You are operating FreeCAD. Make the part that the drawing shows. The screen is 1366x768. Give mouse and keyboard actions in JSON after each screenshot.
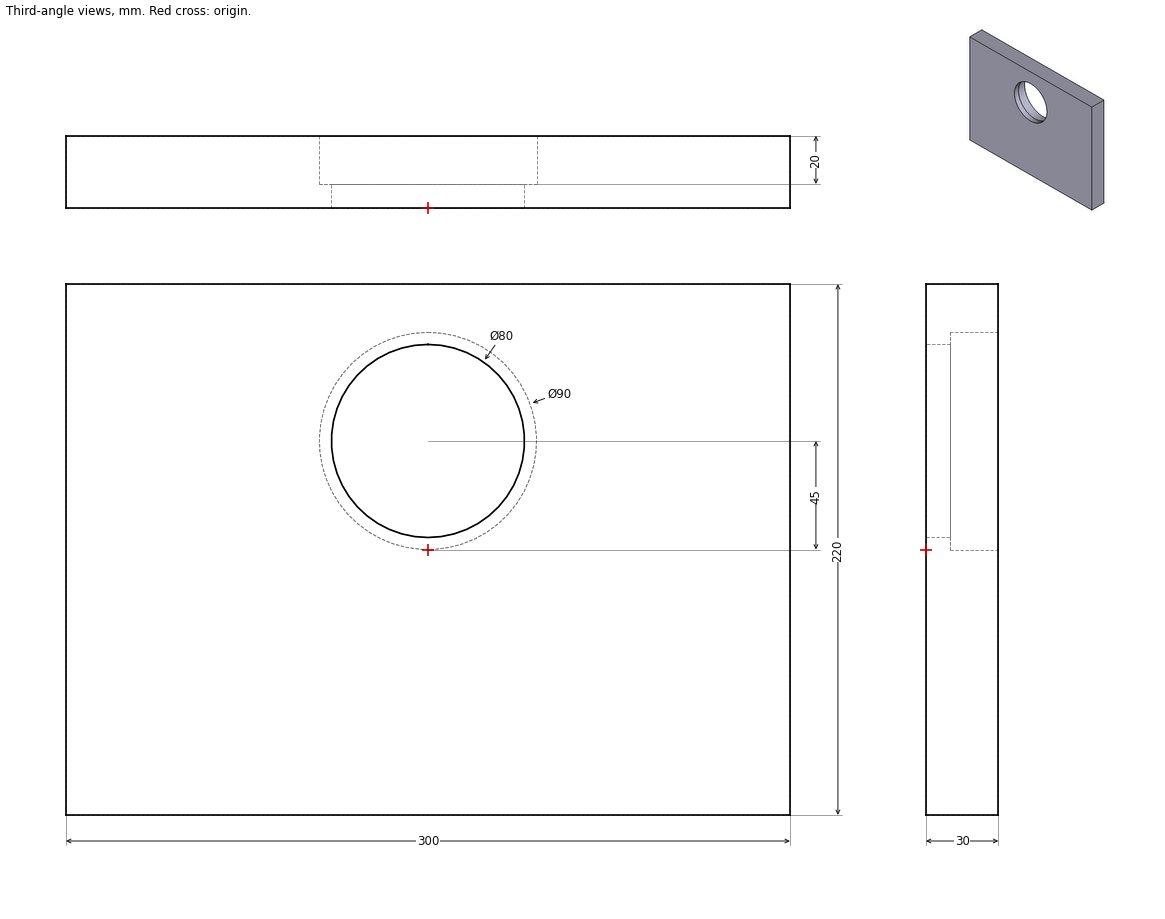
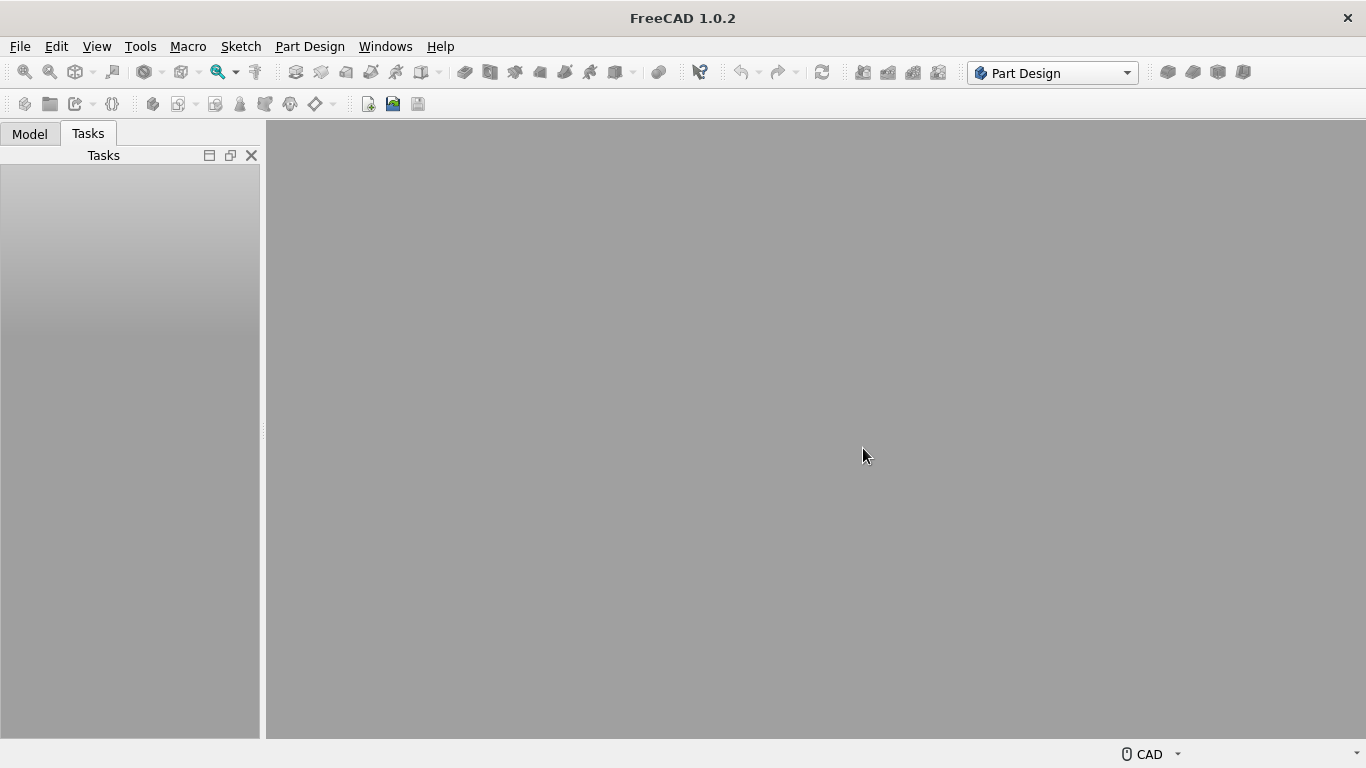
{"action": "left_click", "coordinate": [368, 104]}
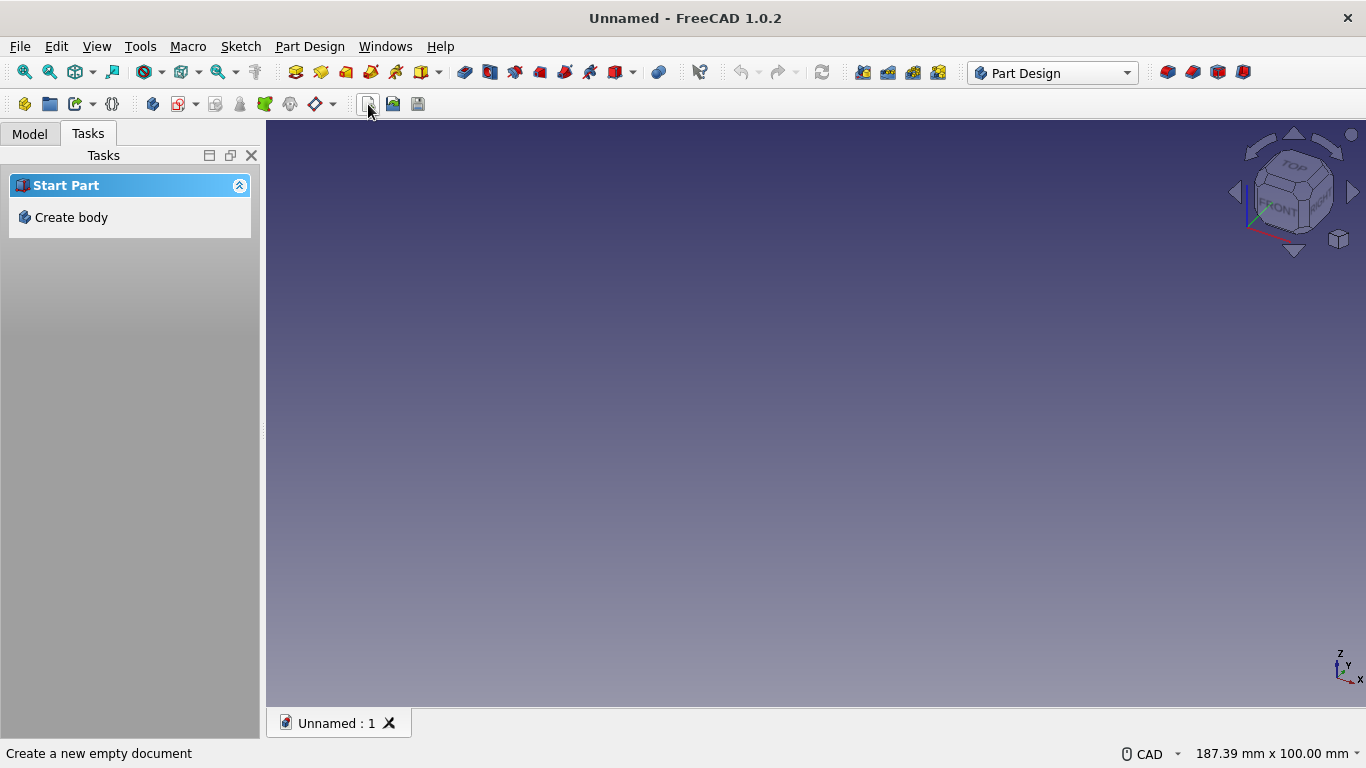
{"action": "left_click", "coordinate": [178, 104]}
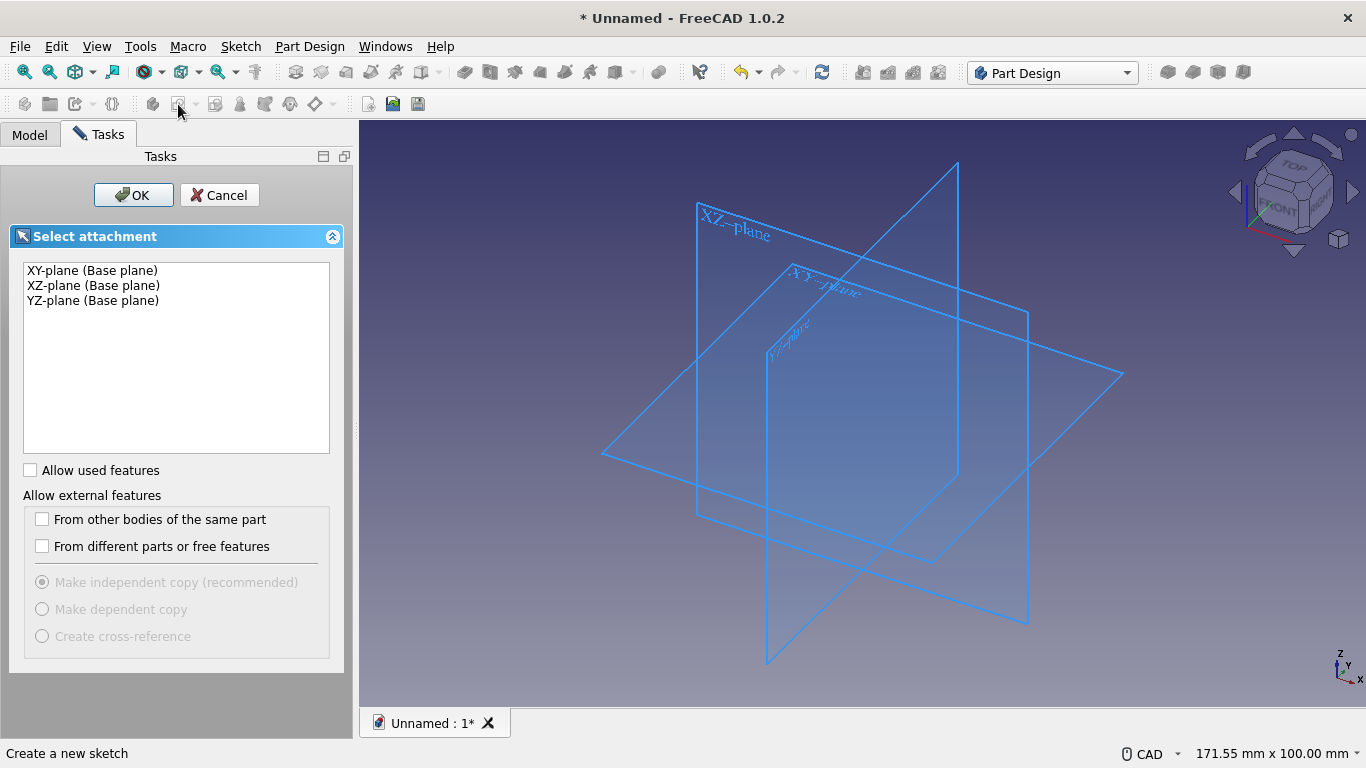
{"action": "left_click", "coordinate": [84, 286]}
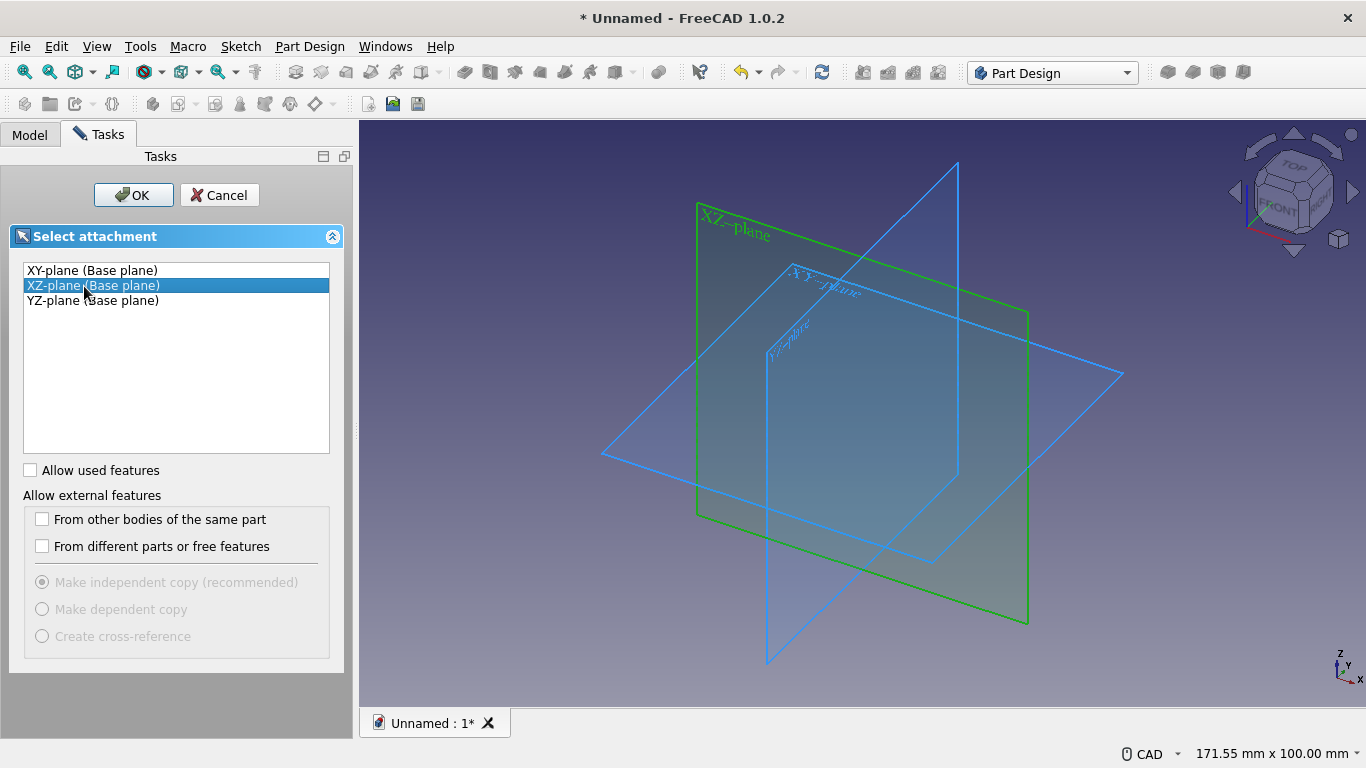
{"action": "left_click", "coordinate": [134, 195]}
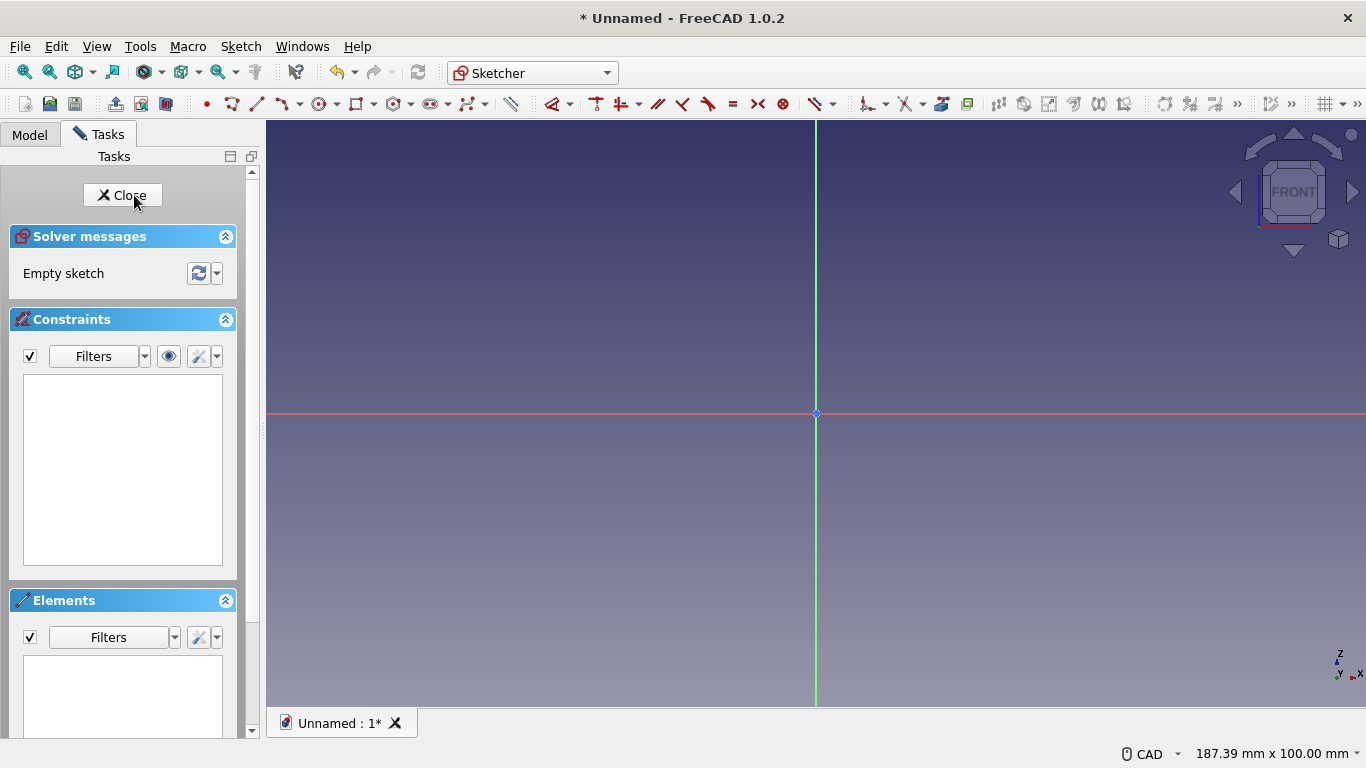
{"action": "scroll", "coordinate": [718, 413], "scroll_direction": "down", "scroll_amount": 6}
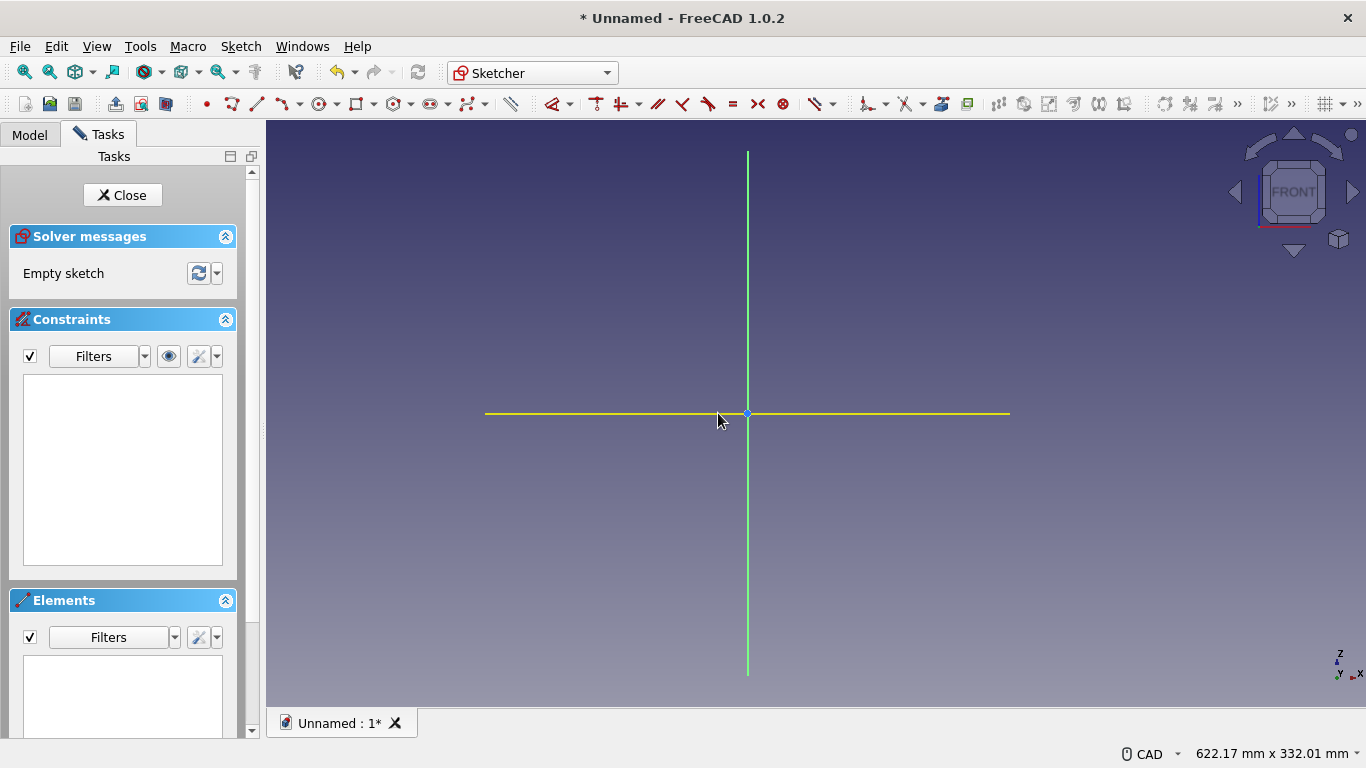
{"action": "key", "text": "g v"}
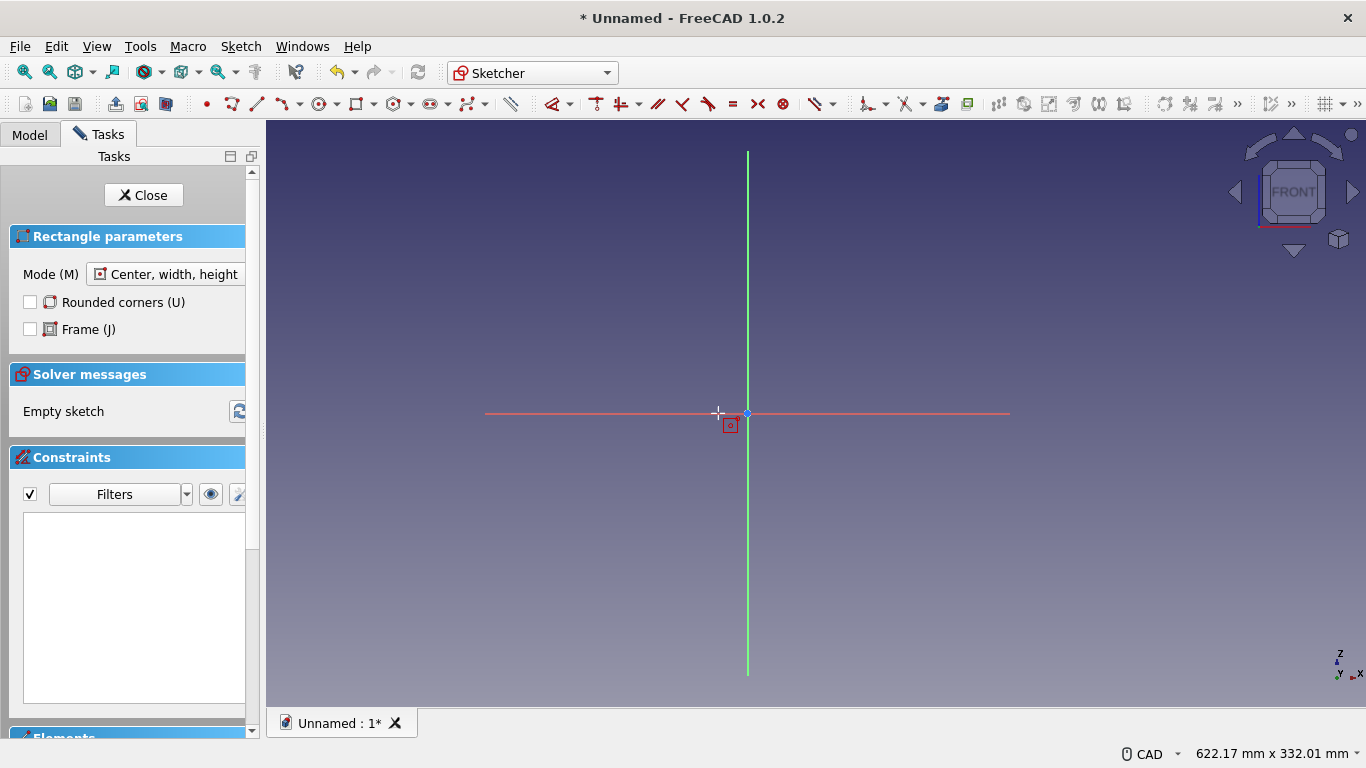
{"action": "left_click", "coordinate": [748, 414]}
{"action": "left_click", "coordinate": [1013, 219]}
{"action": "key", "text": "Escape"}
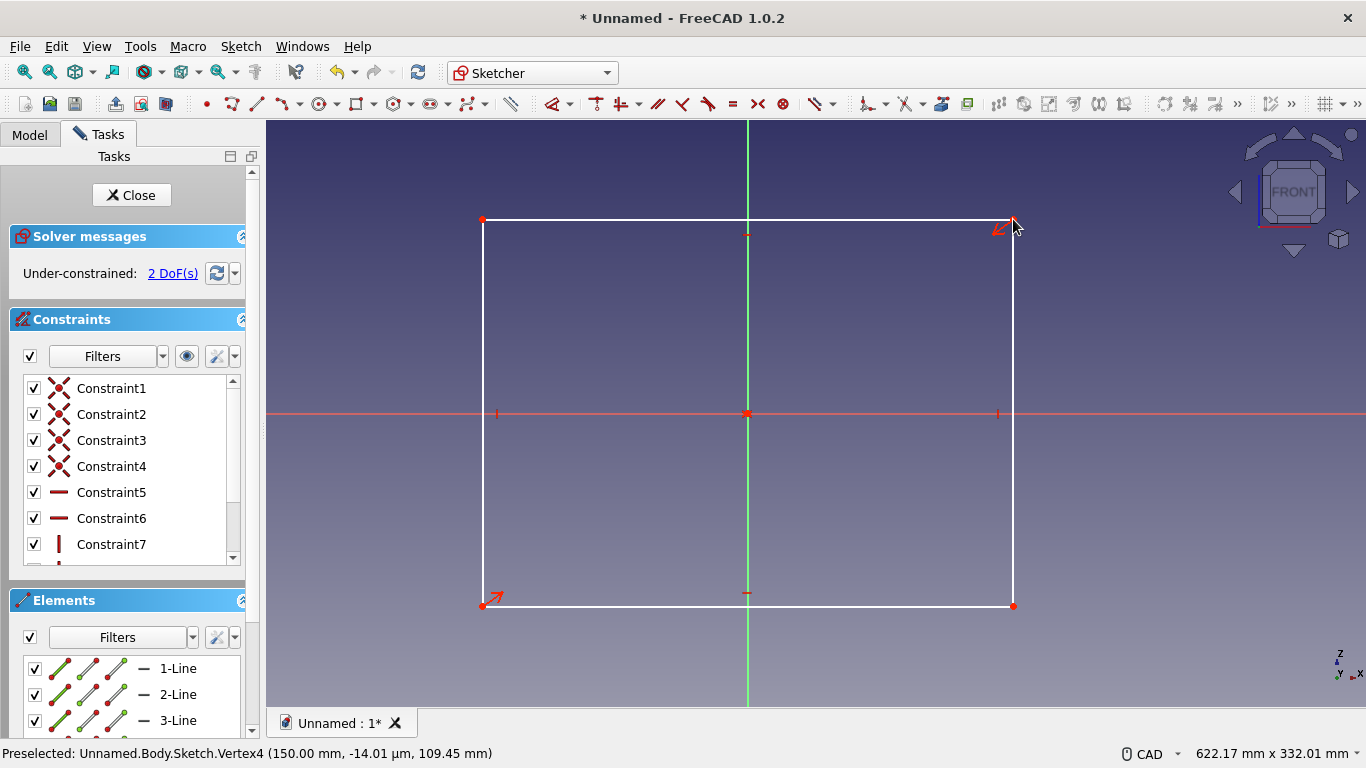
{"action": "left_click", "coordinate": [552, 104]}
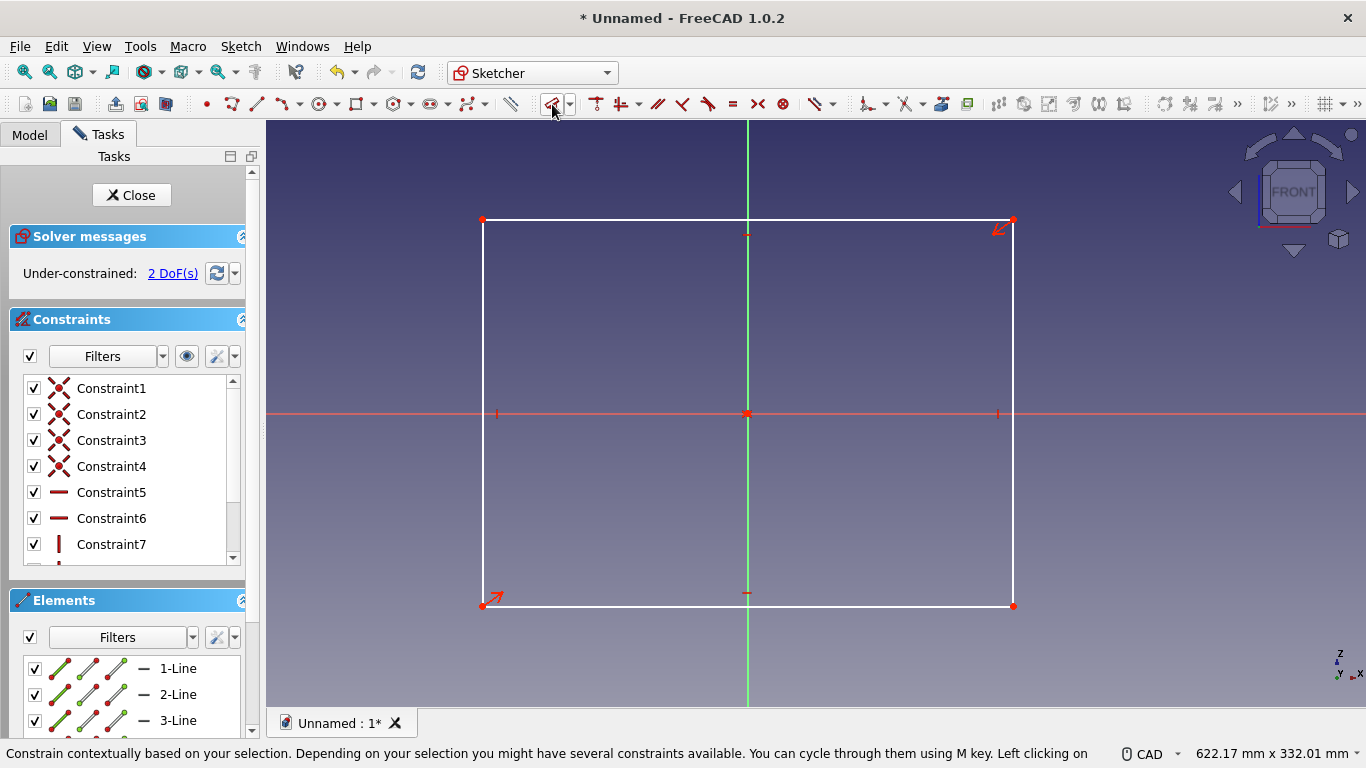
{"action": "left_click", "coordinate": [642, 607]}
{"action": "left_click", "coordinate": [626, 641]}